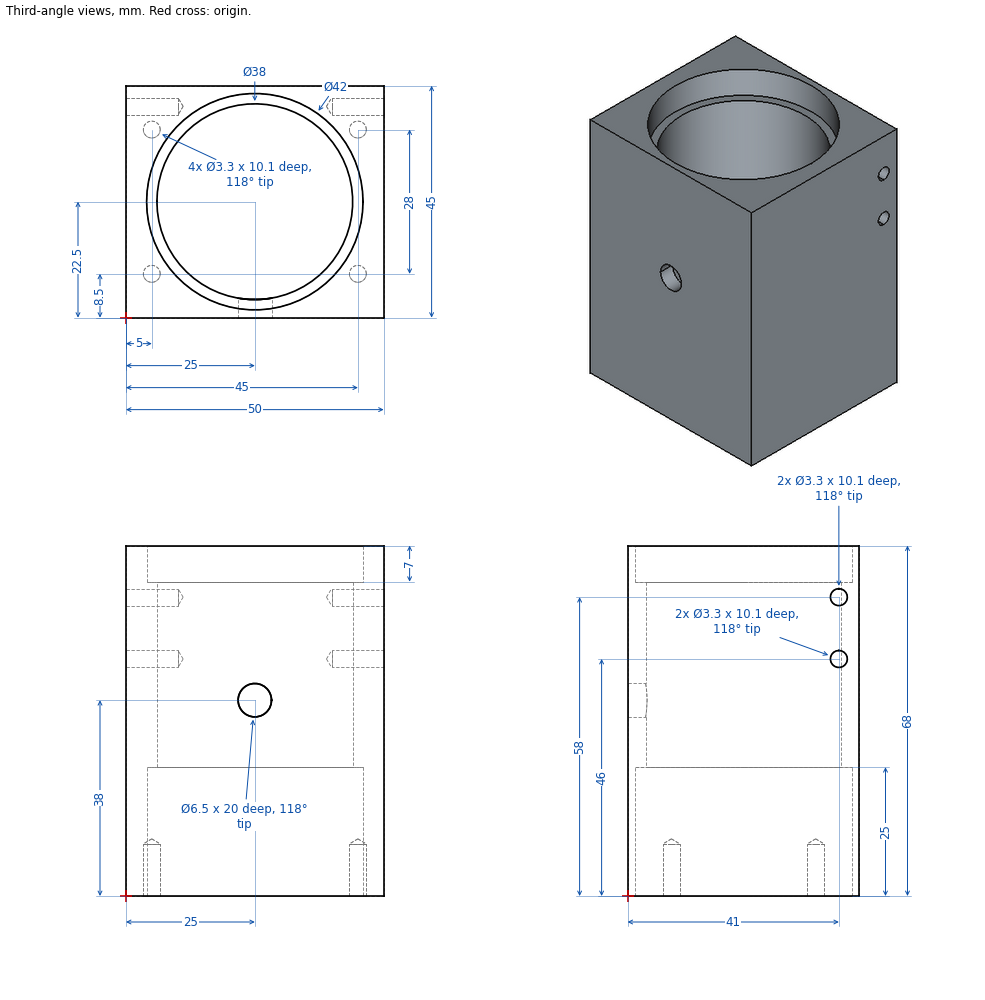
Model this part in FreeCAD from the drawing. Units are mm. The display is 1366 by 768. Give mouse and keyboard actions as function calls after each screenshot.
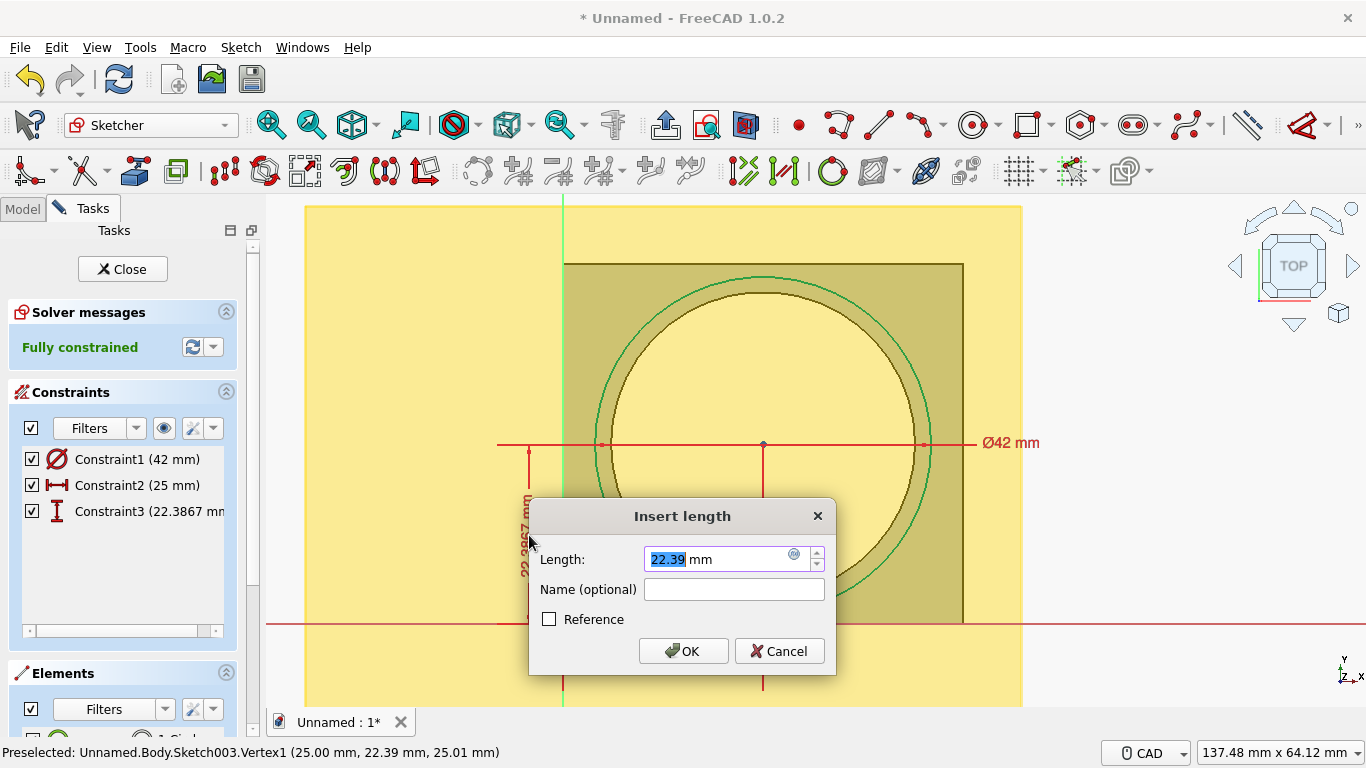
text(22.5)
key(Return)
key(Escape)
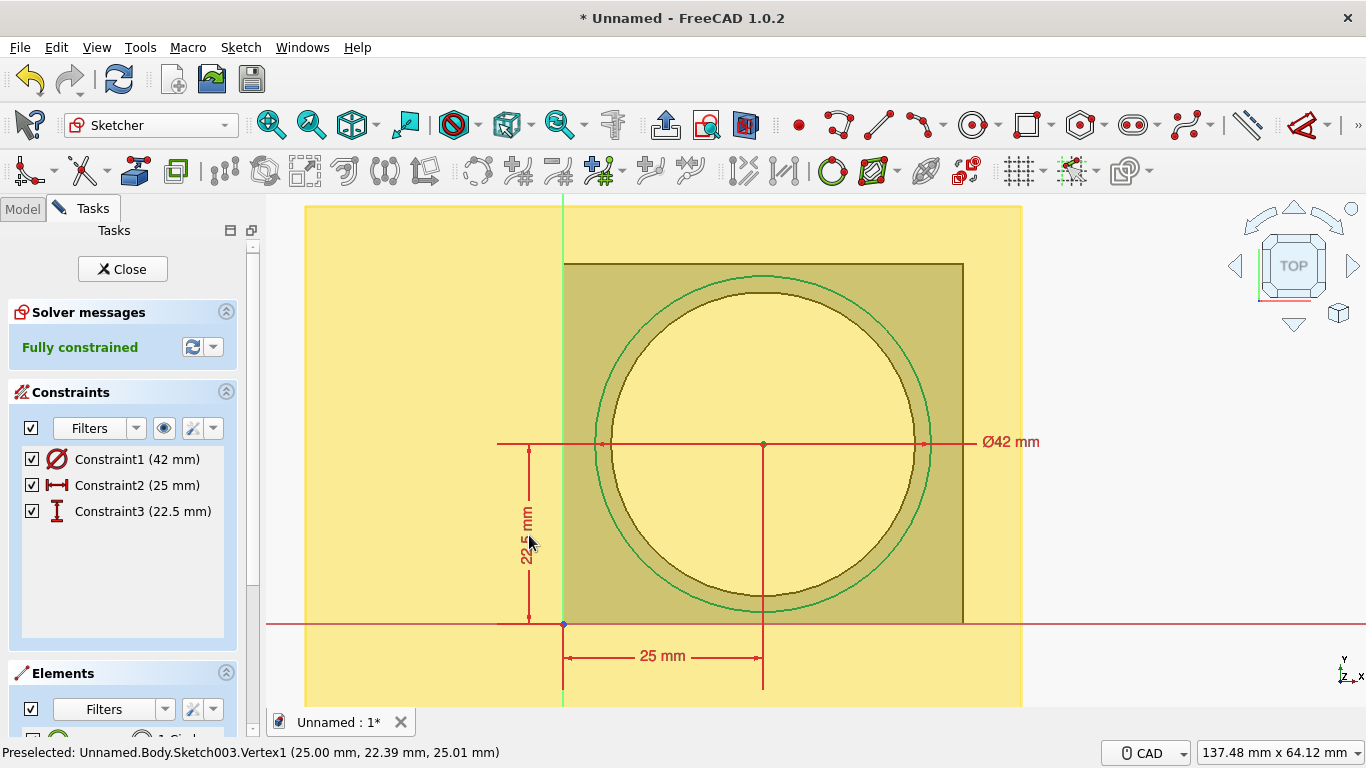
click(123, 269)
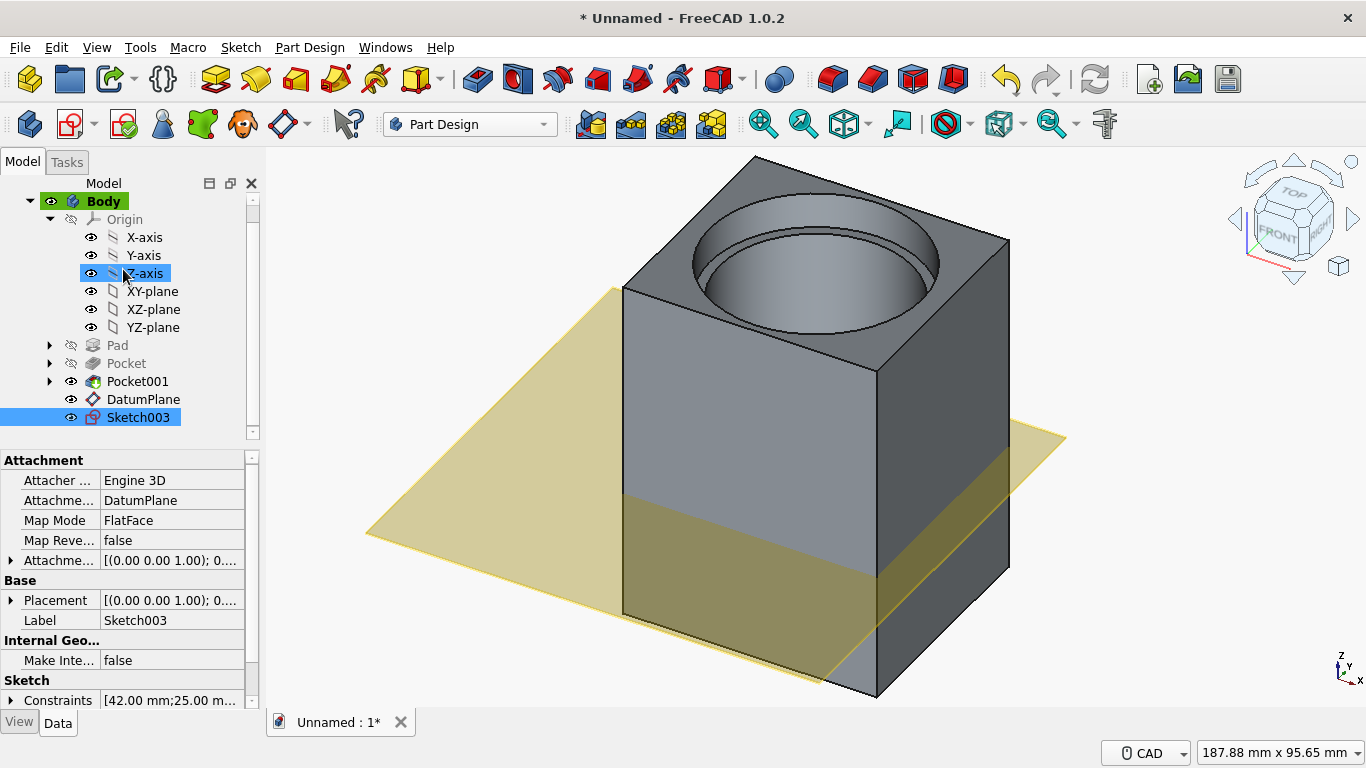
click(478, 80)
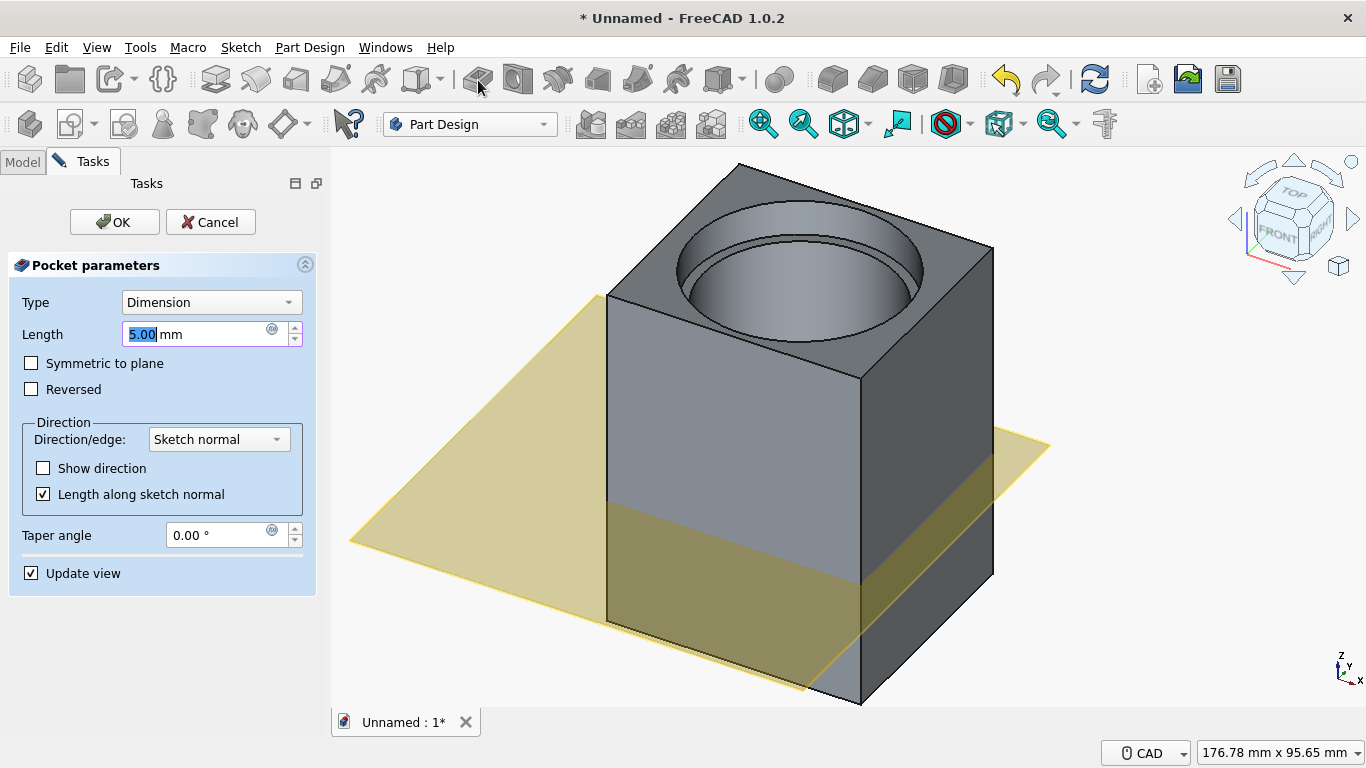
text(25)
key(Tab)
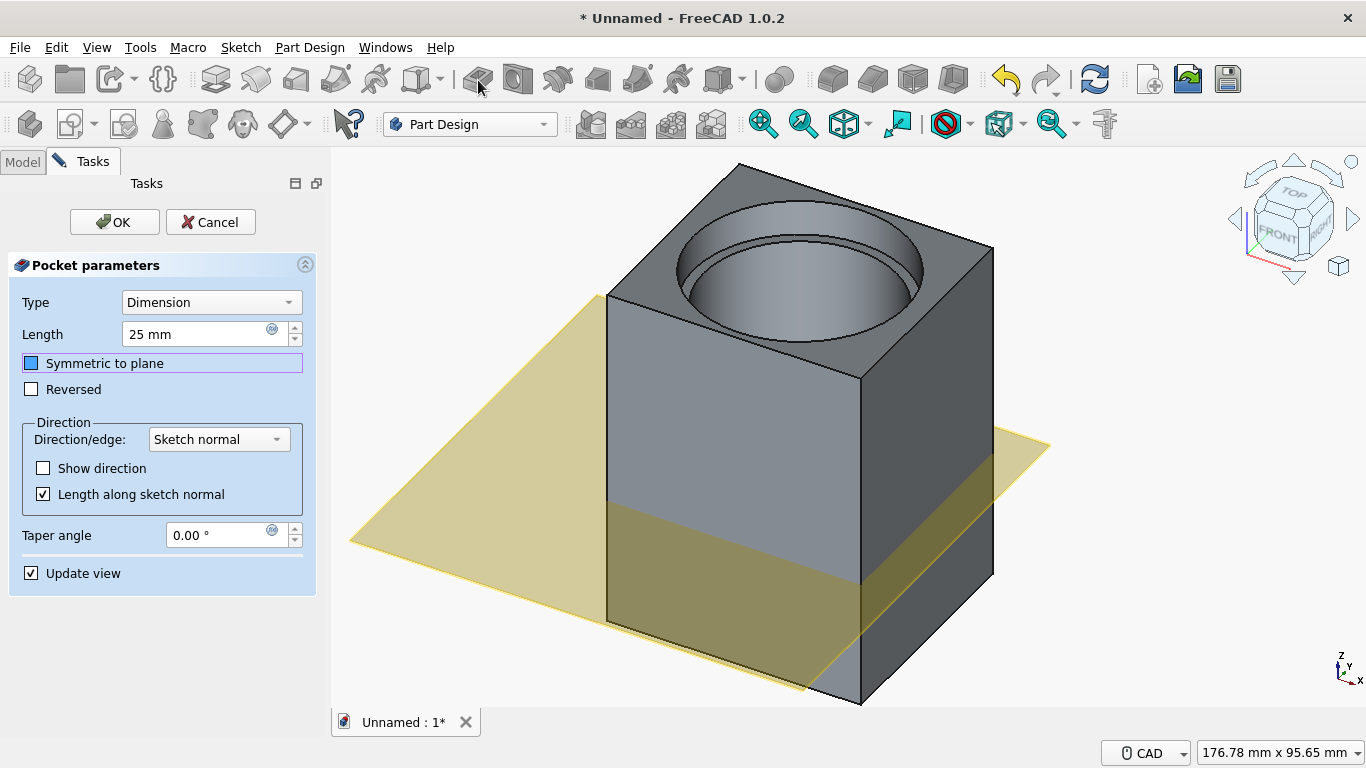
click(115, 222)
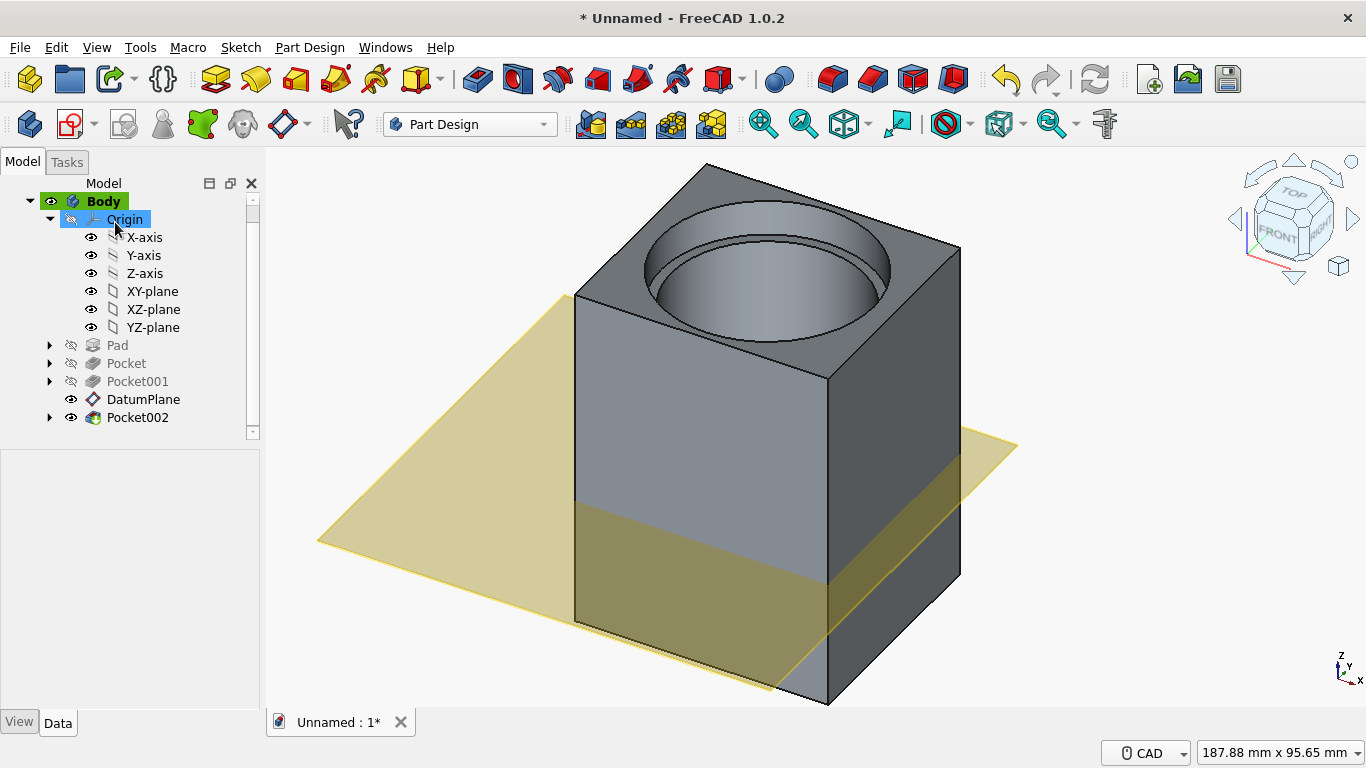
click(116, 399)
key(space)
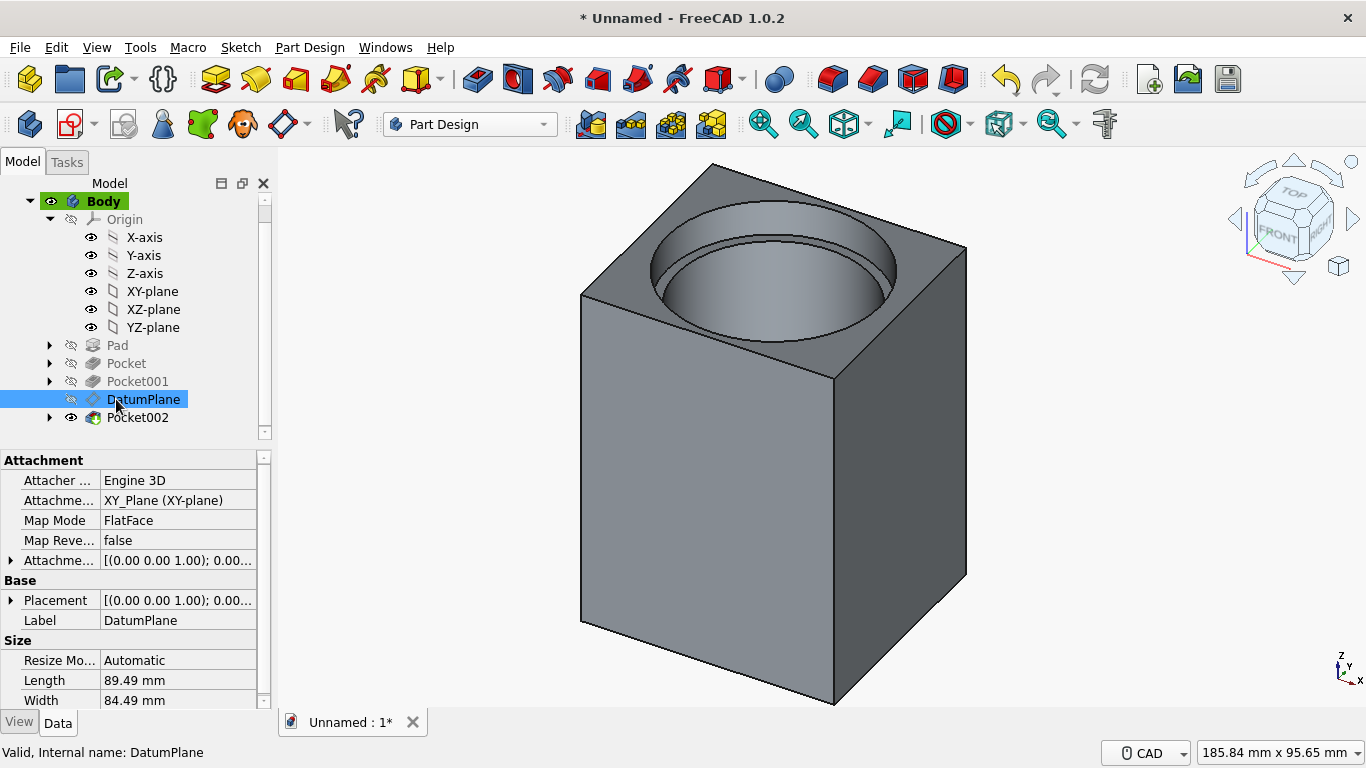
click(900, 429)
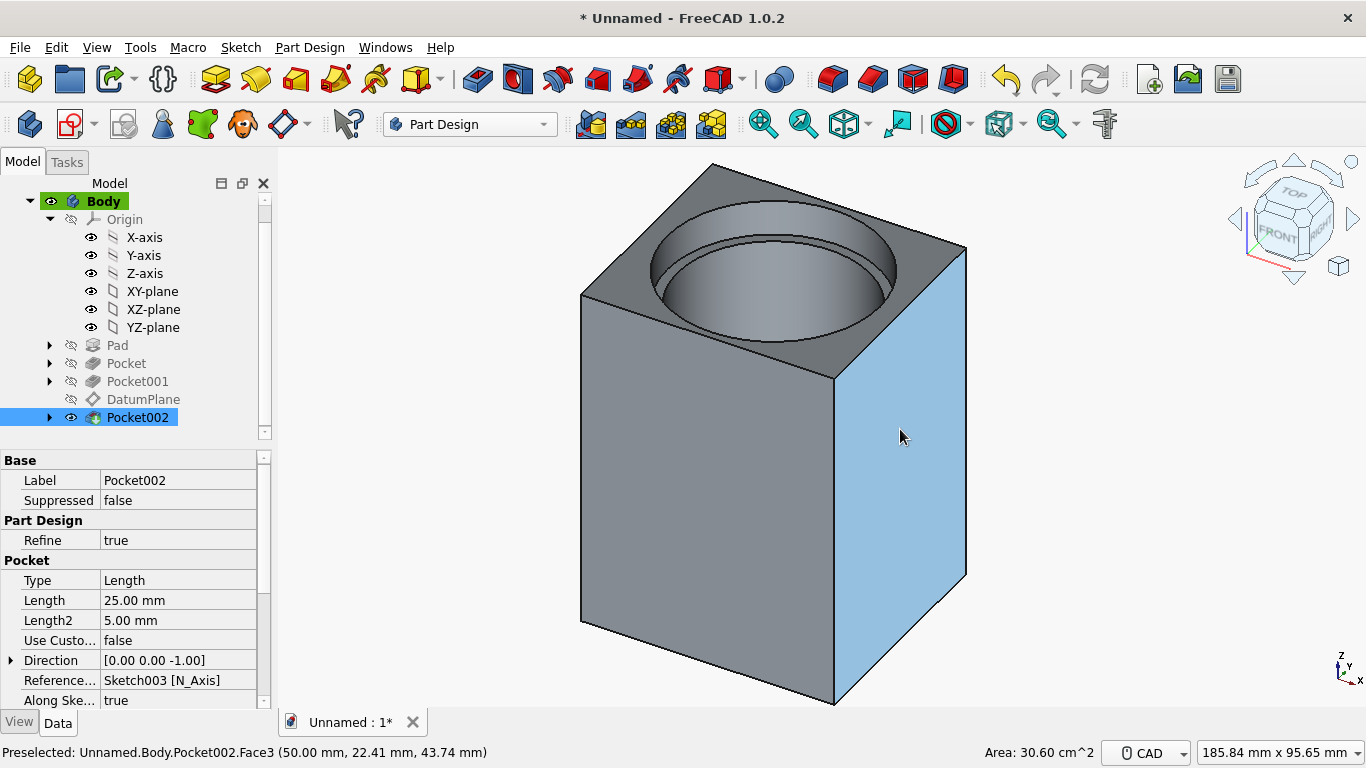
click(70, 124)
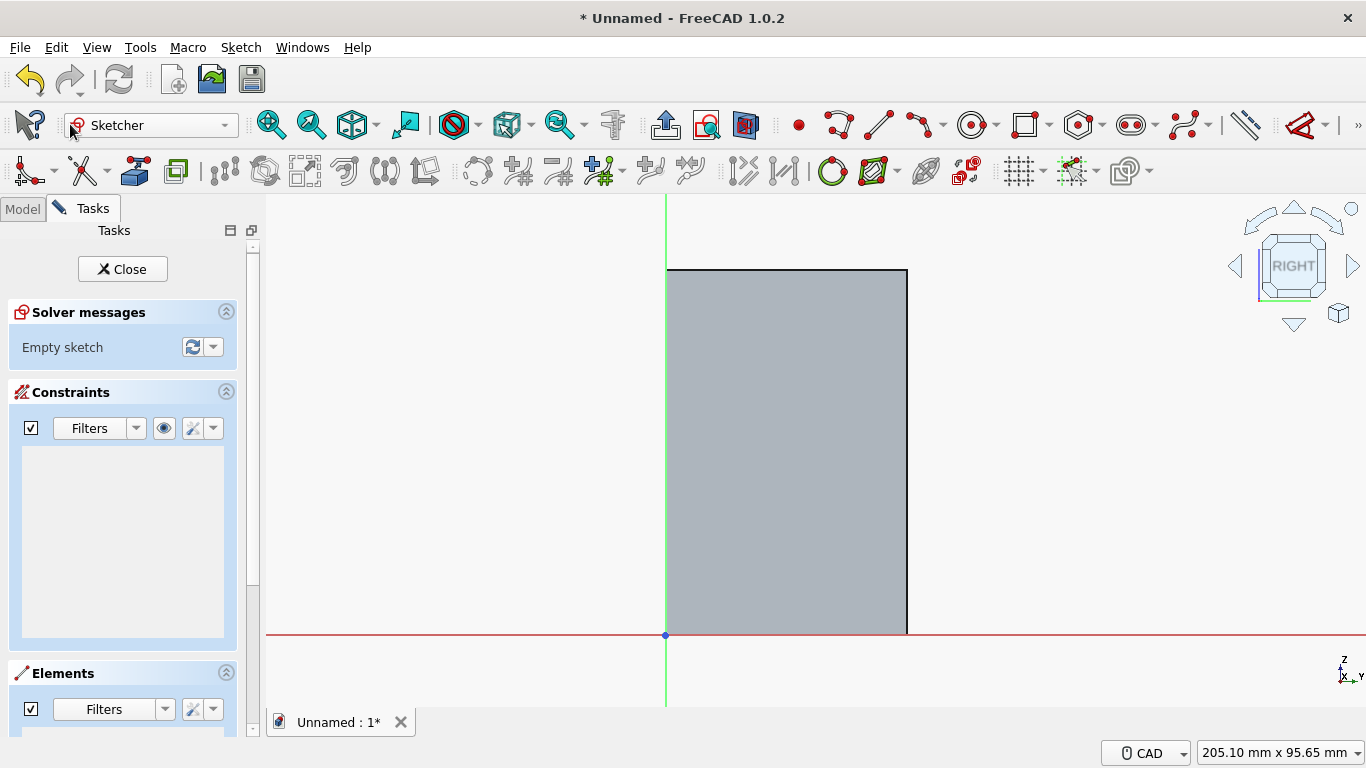
scroll(931, 325, up, 7)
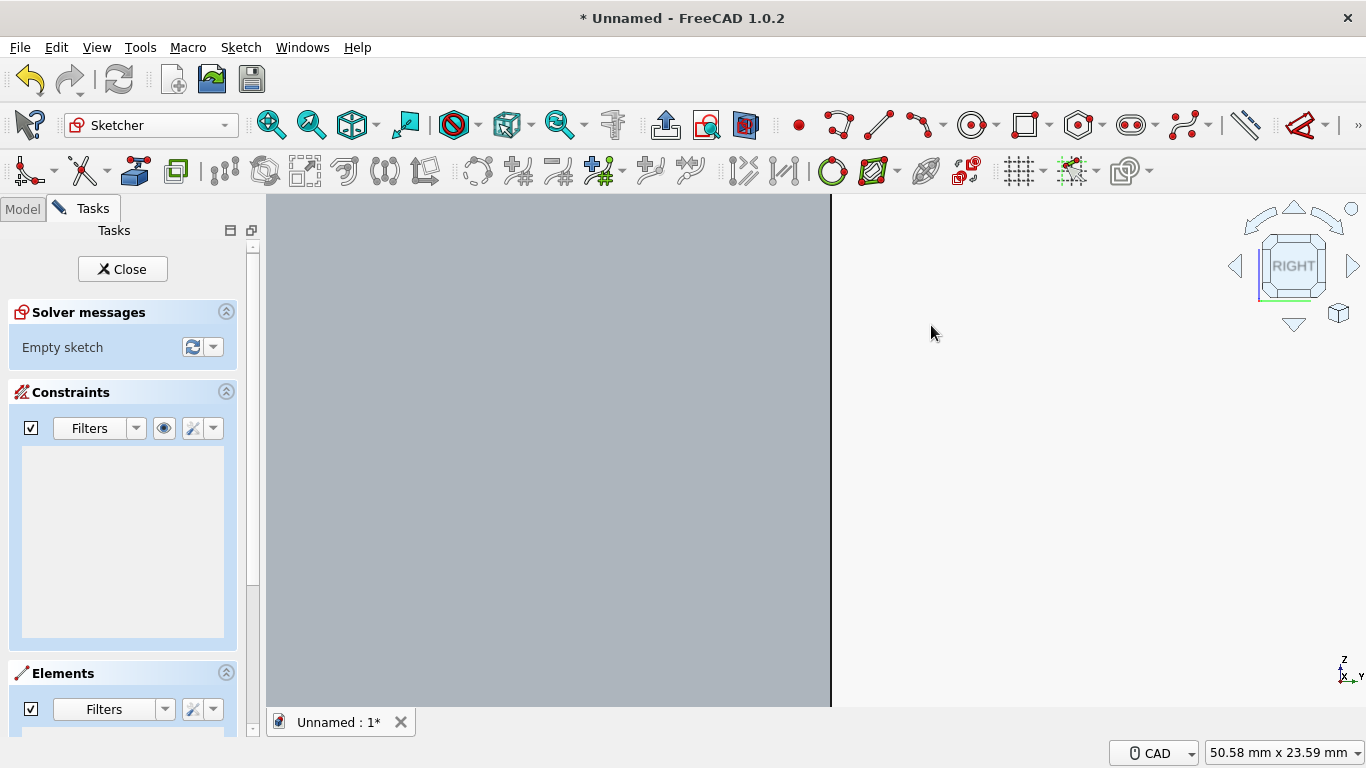
click(972, 126)